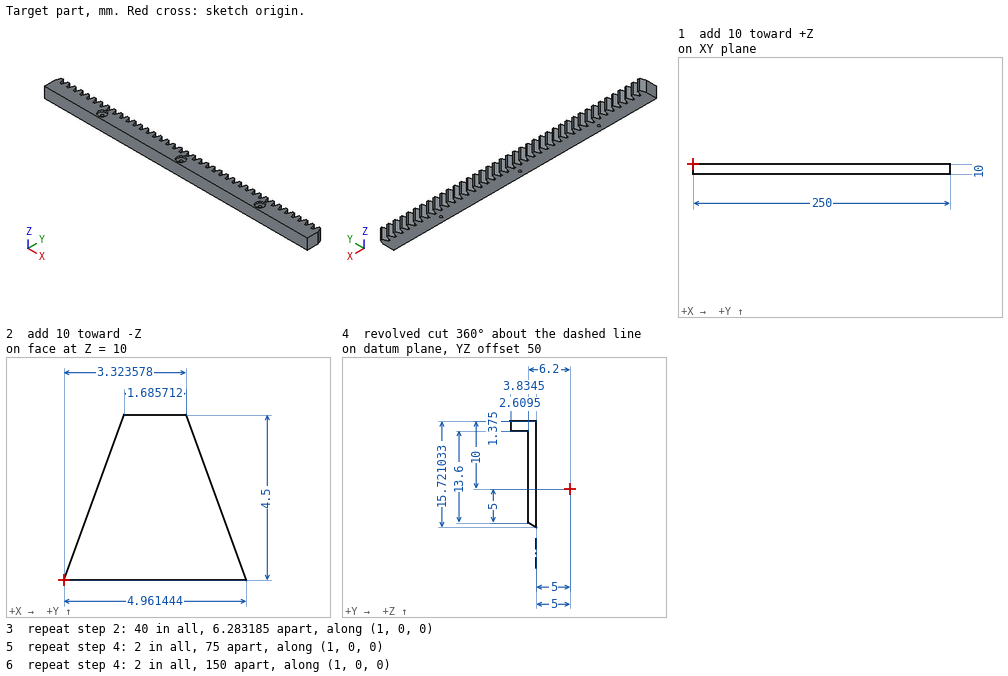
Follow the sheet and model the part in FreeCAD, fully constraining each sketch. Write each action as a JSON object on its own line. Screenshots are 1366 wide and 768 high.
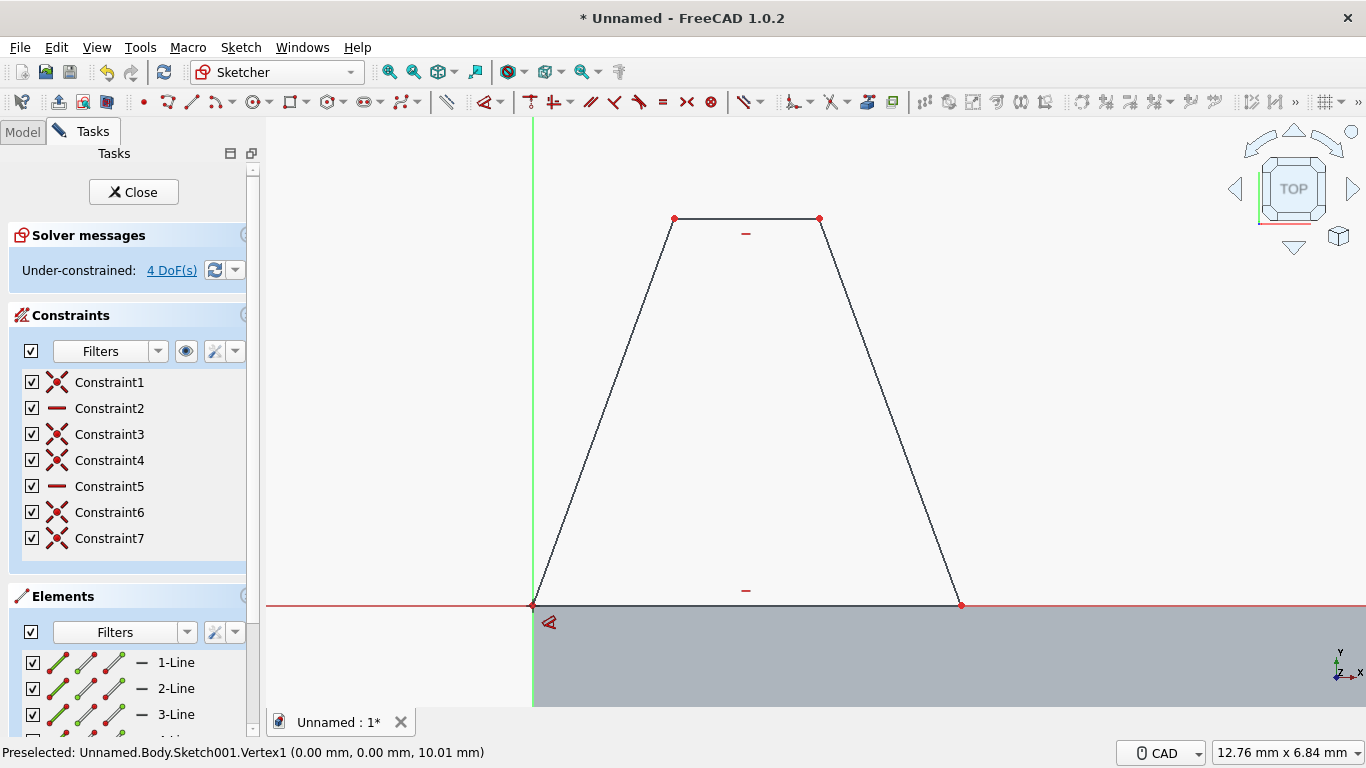
{"action": "left_click", "coordinate": [819, 219]}
{"action": "left_click", "coordinate": [499, 412]}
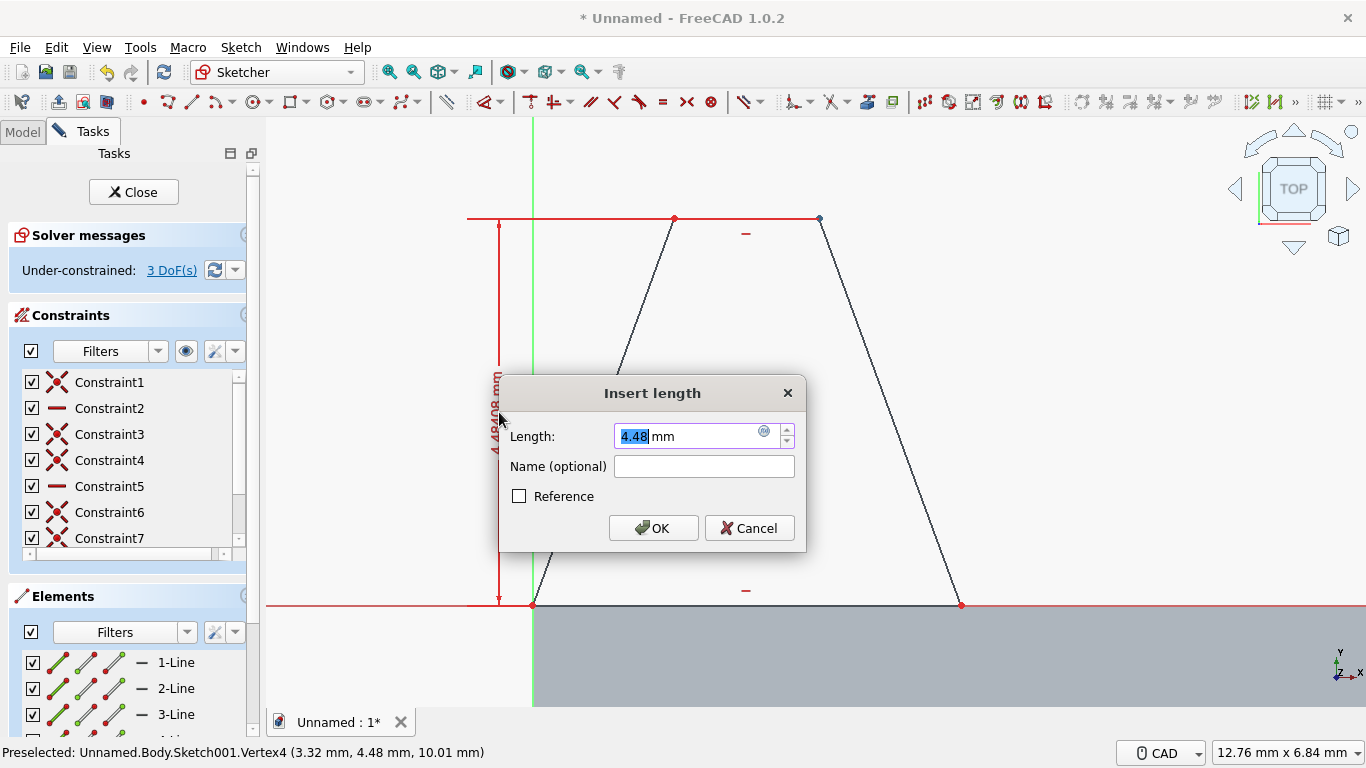
{"action": "type", "text": "4.5"}
{"action": "key", "text": "Return"}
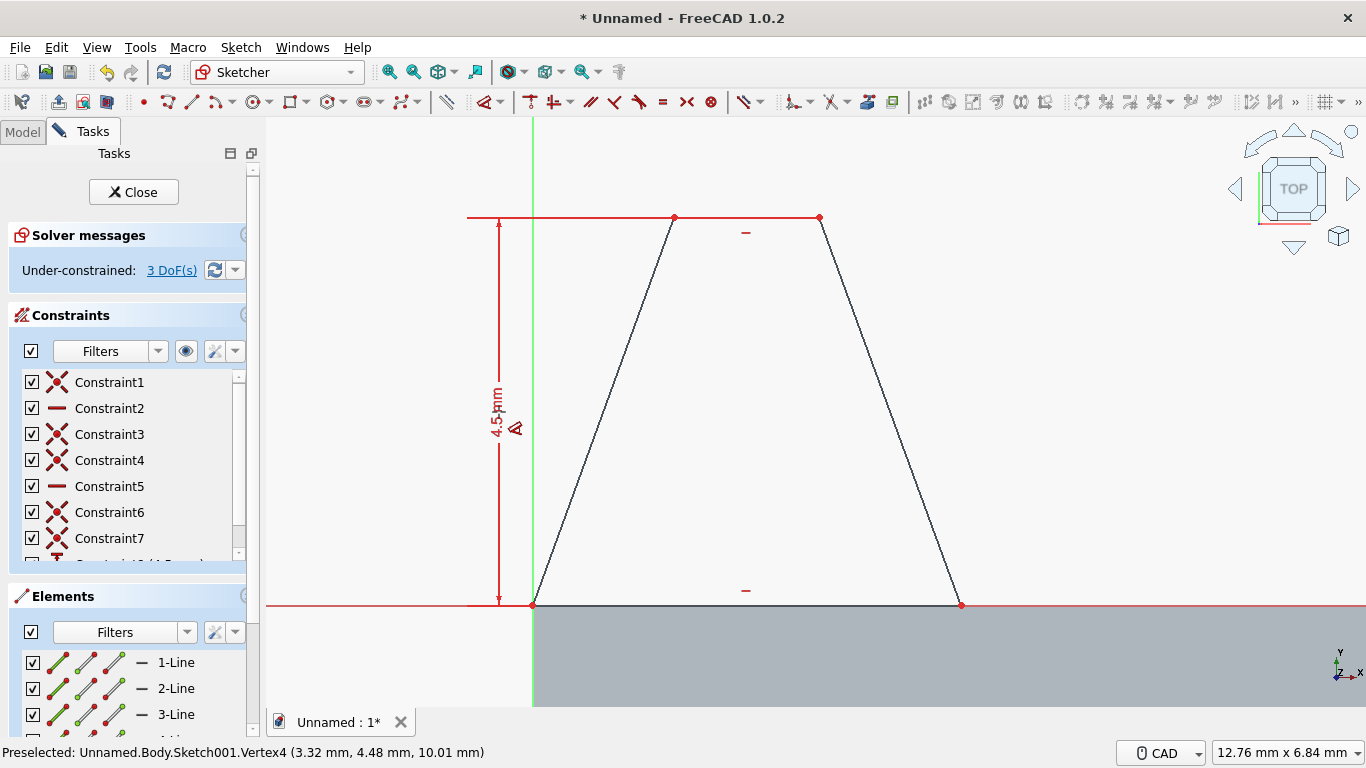
{"action": "left_click", "coordinate": [661, 606]}
{"action": "left_click", "coordinate": [747, 640]}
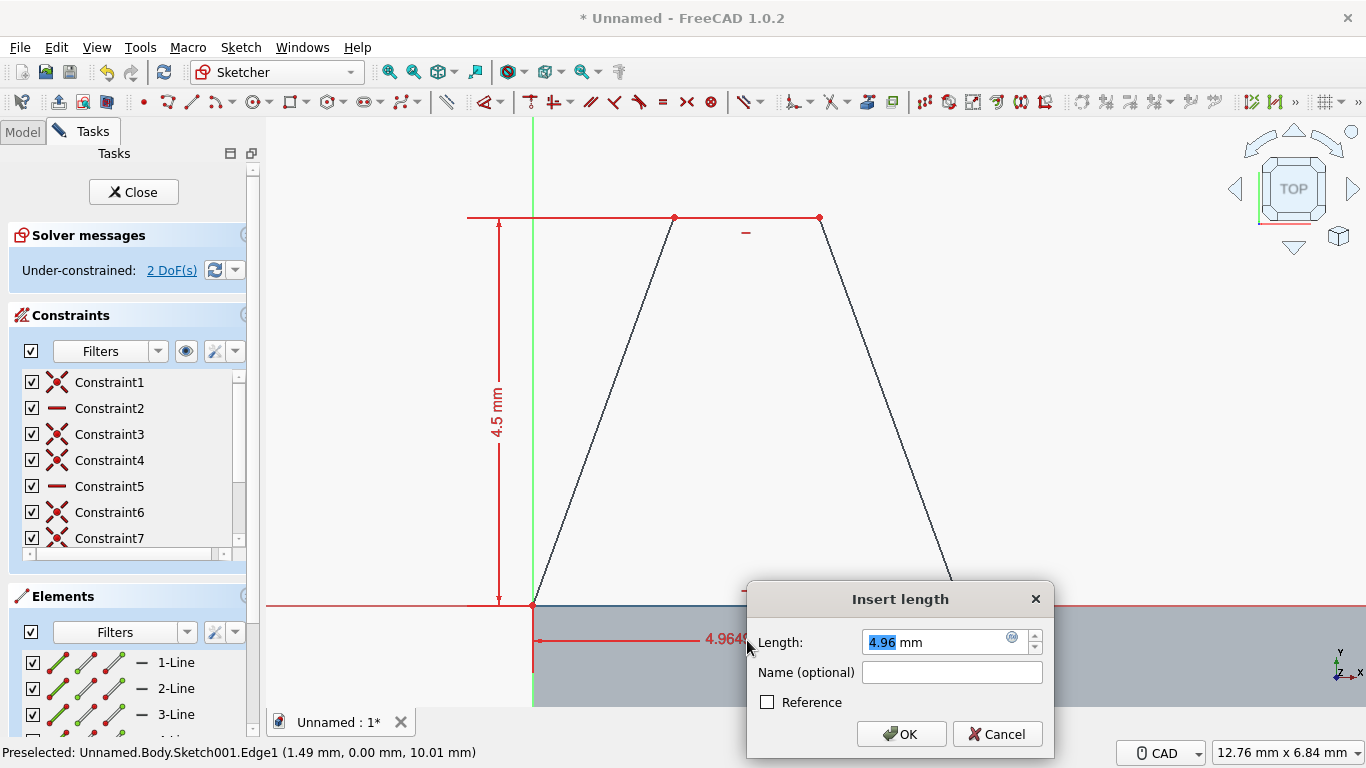
{"action": "type", "text": "4.961444"}
{"action": "key", "text": "Return"}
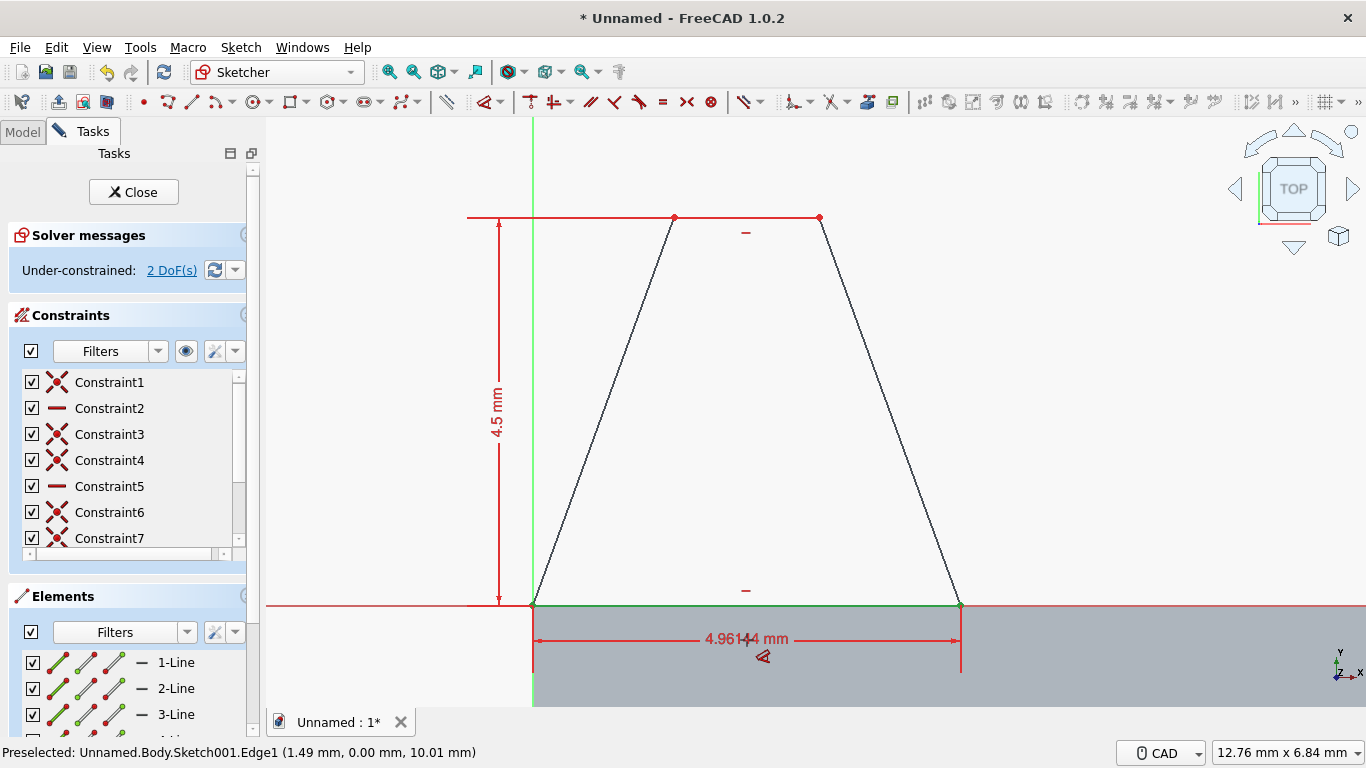
{"action": "left_click", "coordinate": [776, 218]}
{"action": "left_click", "coordinate": [747, 184]}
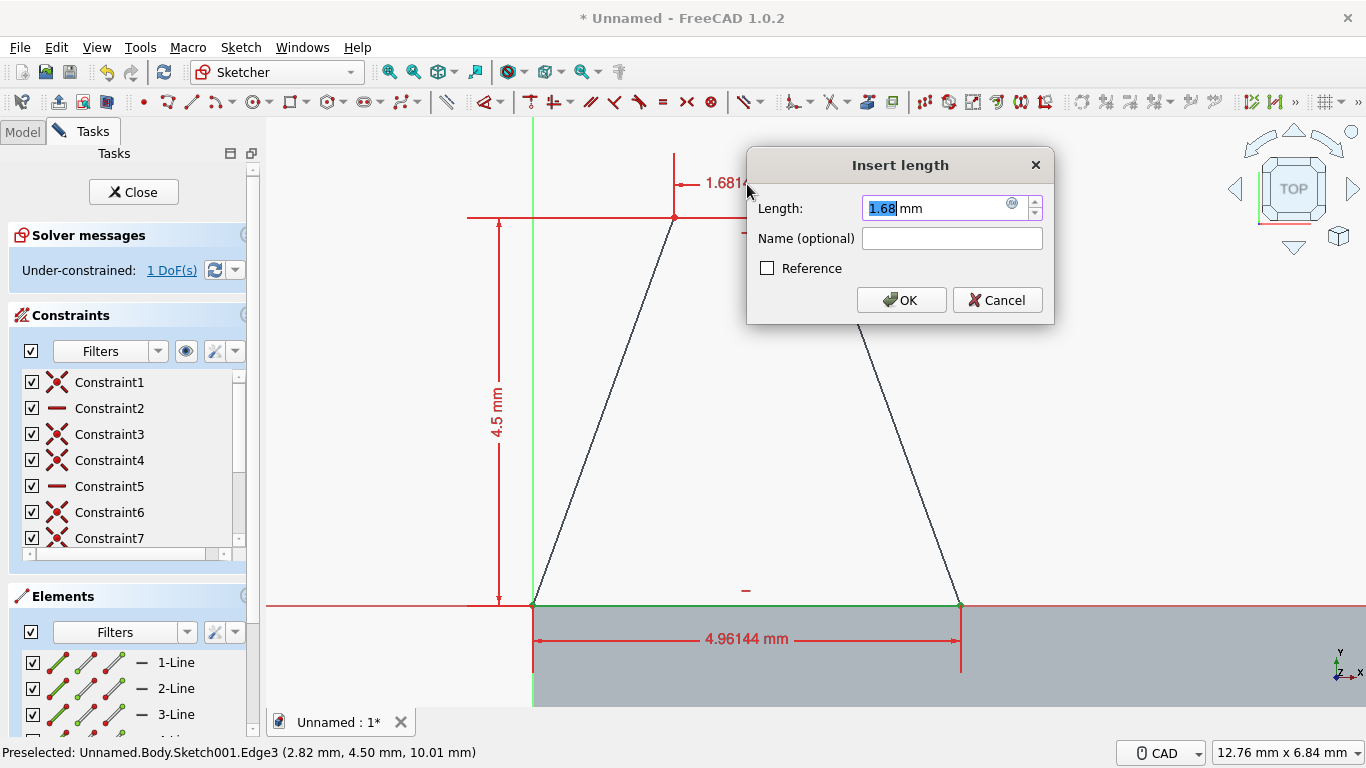
{"action": "type", "text": "1.685712"}
{"action": "key", "text": "Return"}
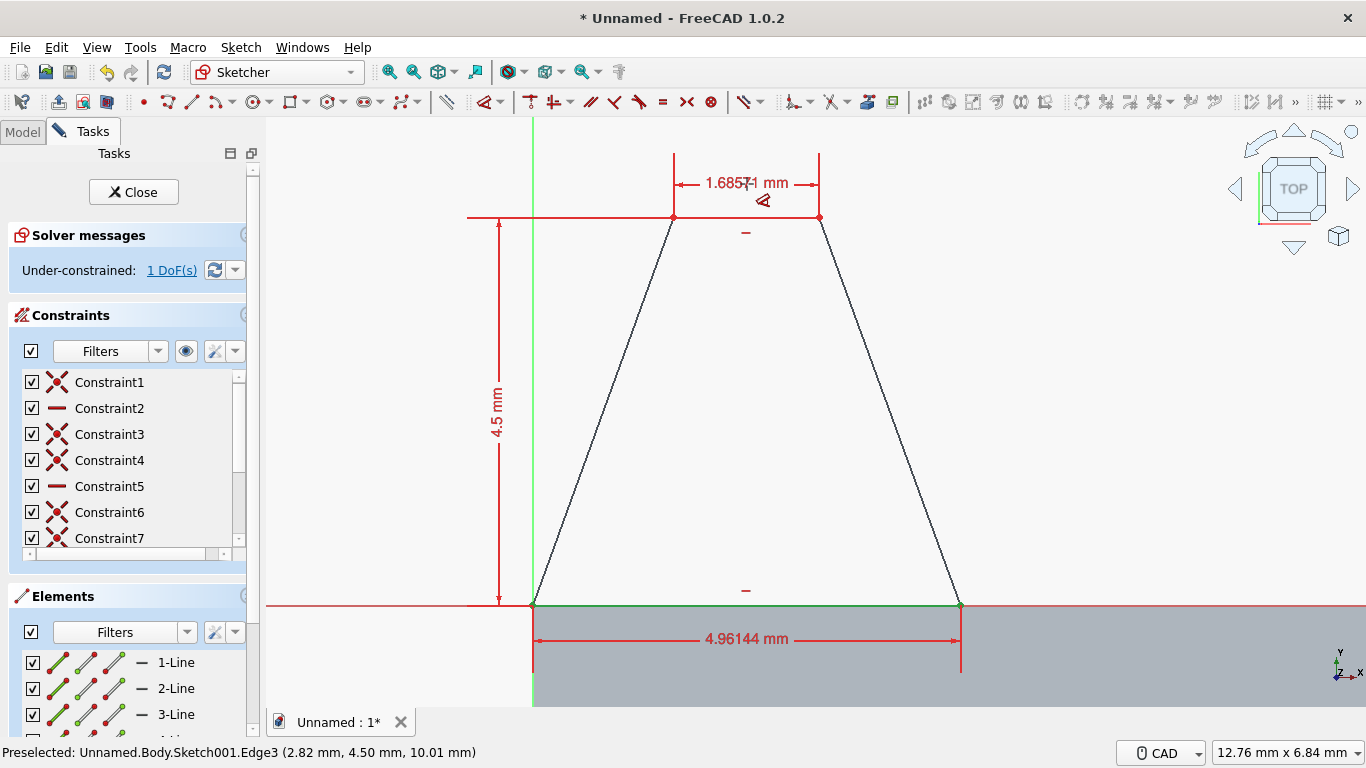
{"action": "left_click", "coordinate": [819, 218]}
{"action": "left_click", "coordinate": [676, 640]}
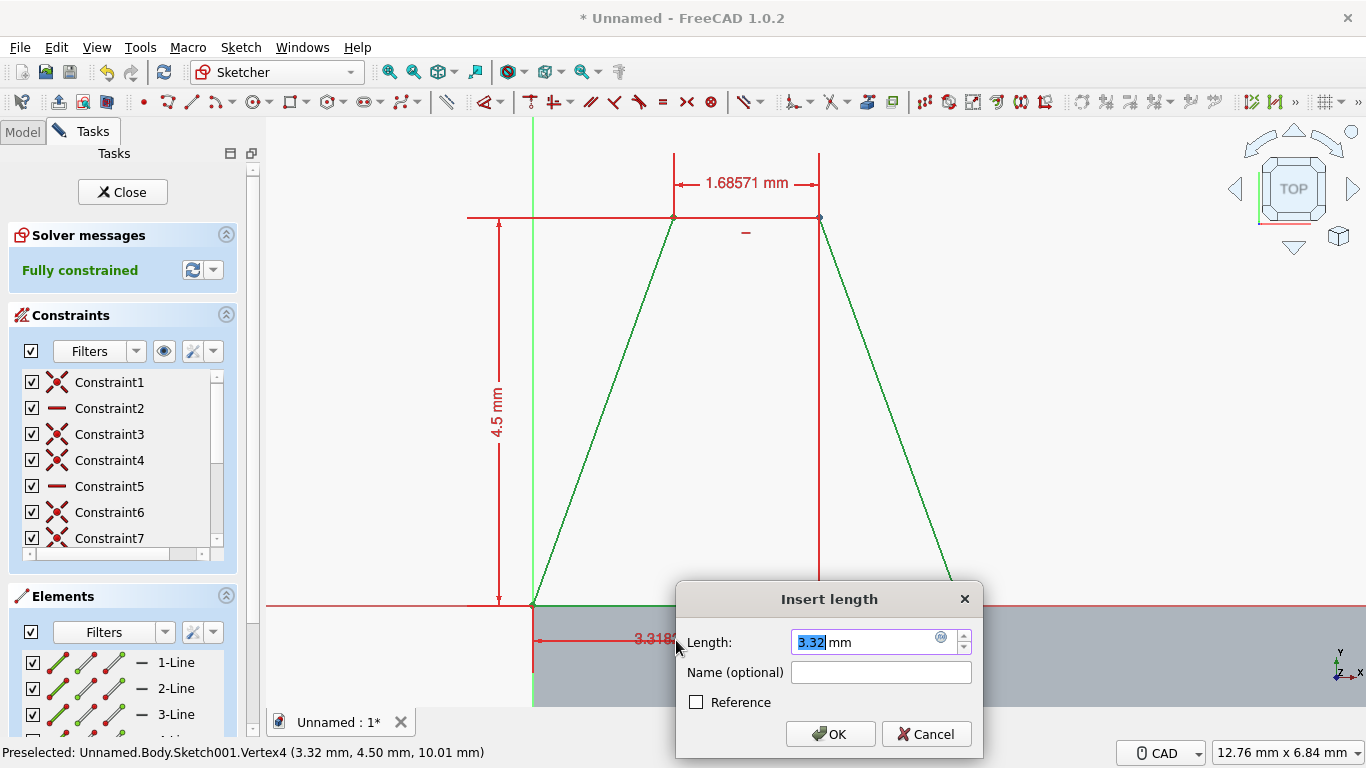
{"action": "type", "text": "3.323578"}
{"action": "key", "text": "Return"}
{"action": "key", "text": "Escape"}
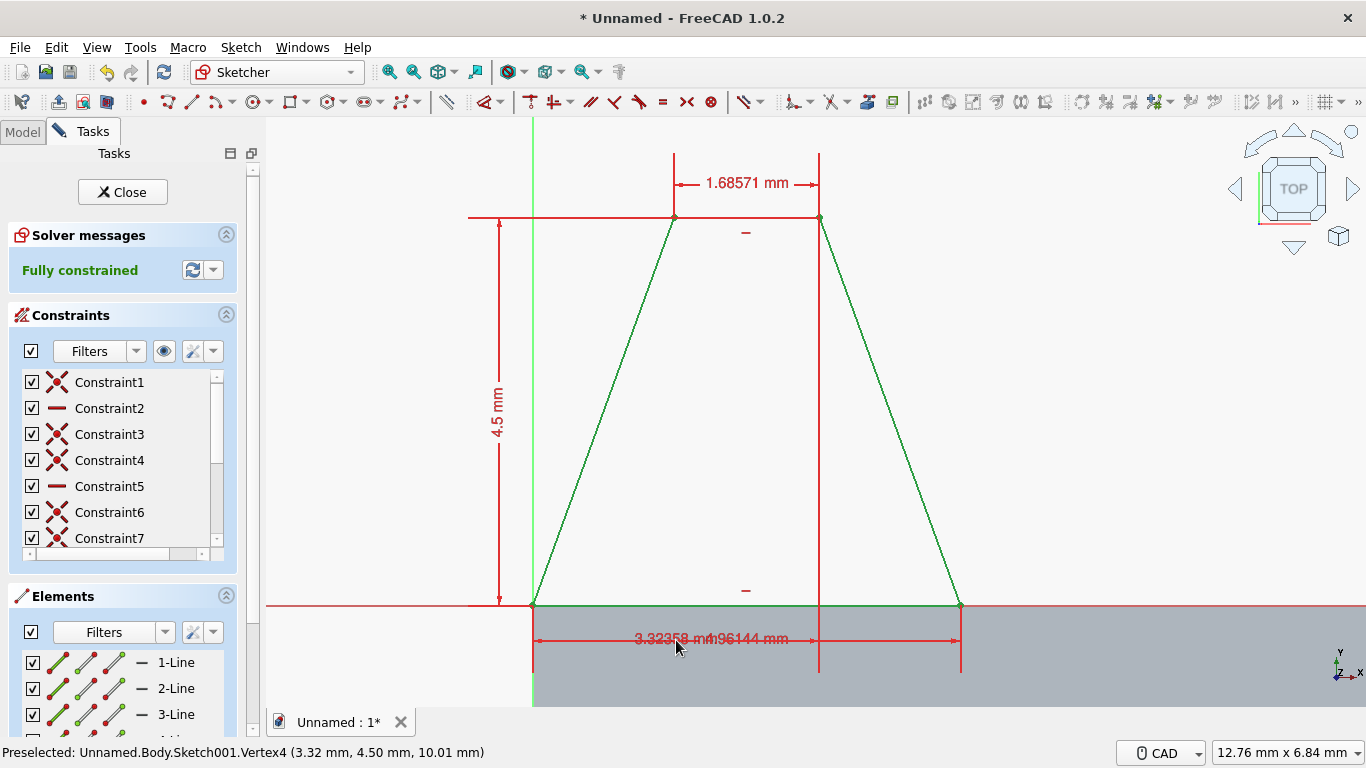
{"action": "left_click", "coordinate": [123, 192]}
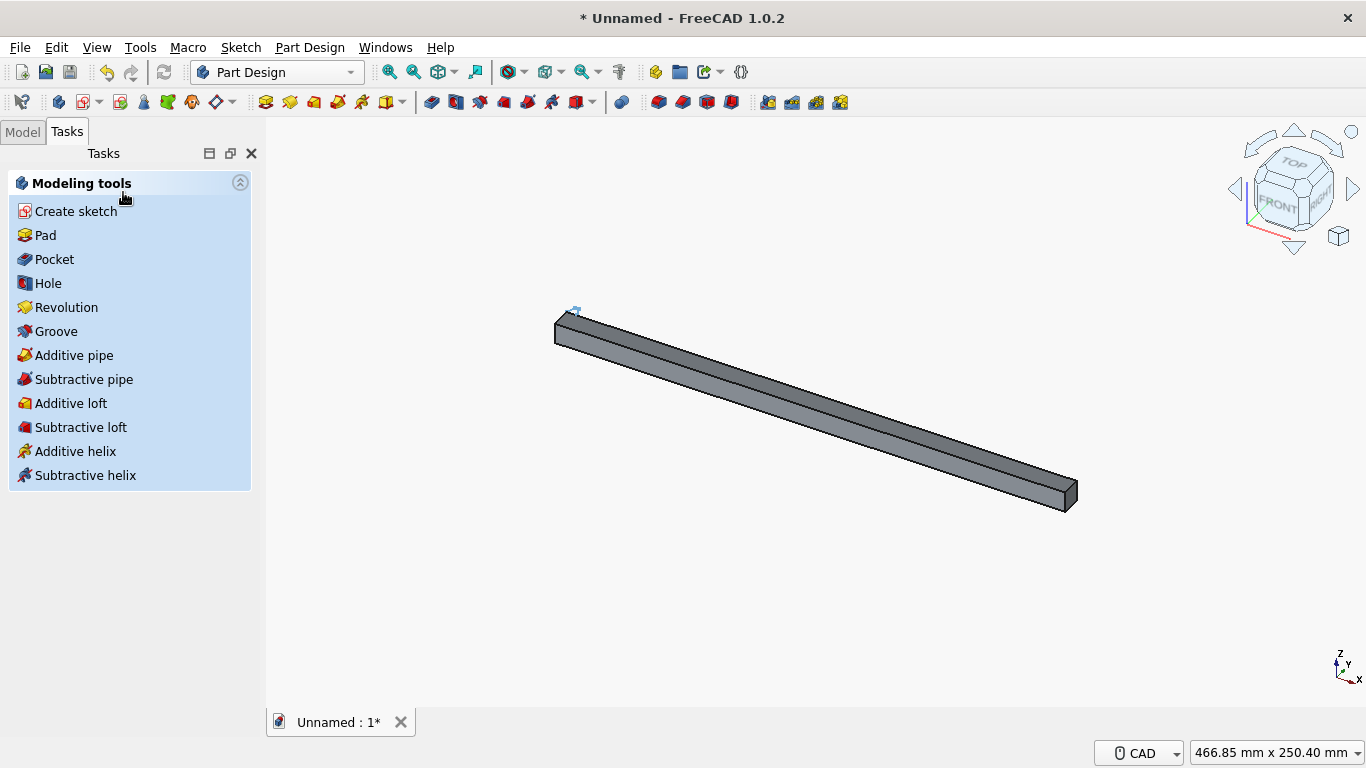
{"action": "left_click", "coordinate": [266, 102]}